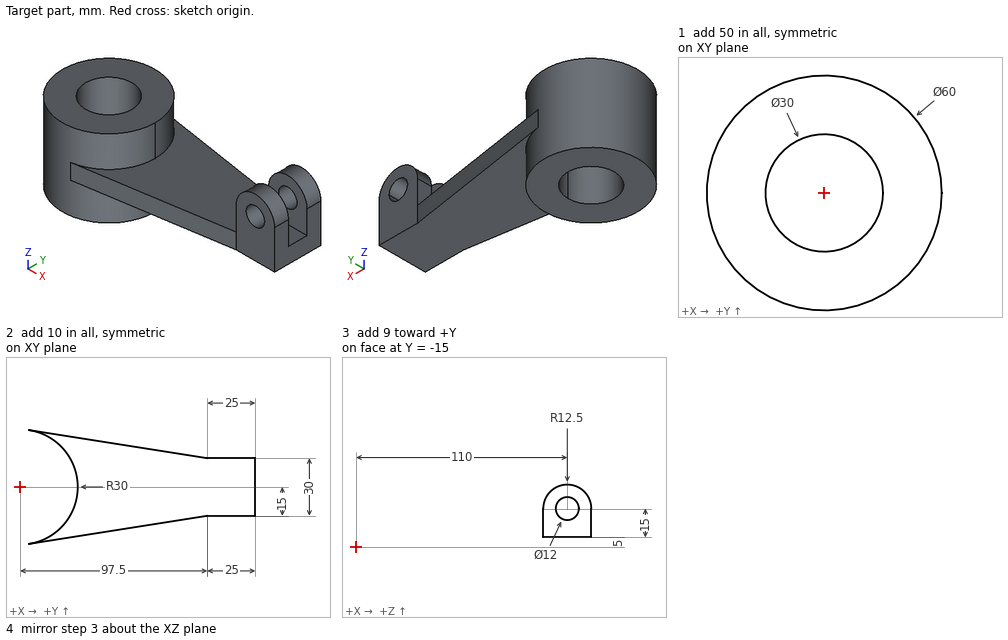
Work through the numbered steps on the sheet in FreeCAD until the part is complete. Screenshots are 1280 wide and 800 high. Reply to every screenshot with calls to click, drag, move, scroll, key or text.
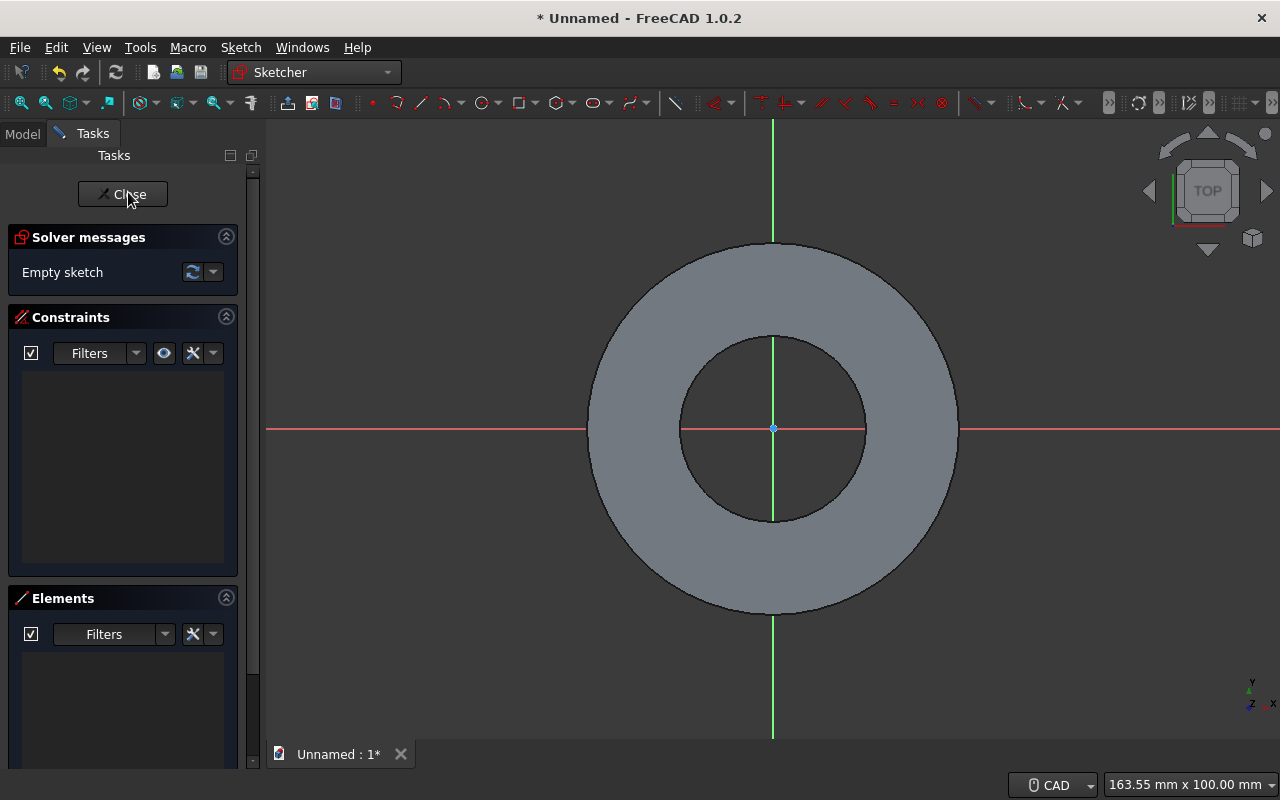
click(336, 104)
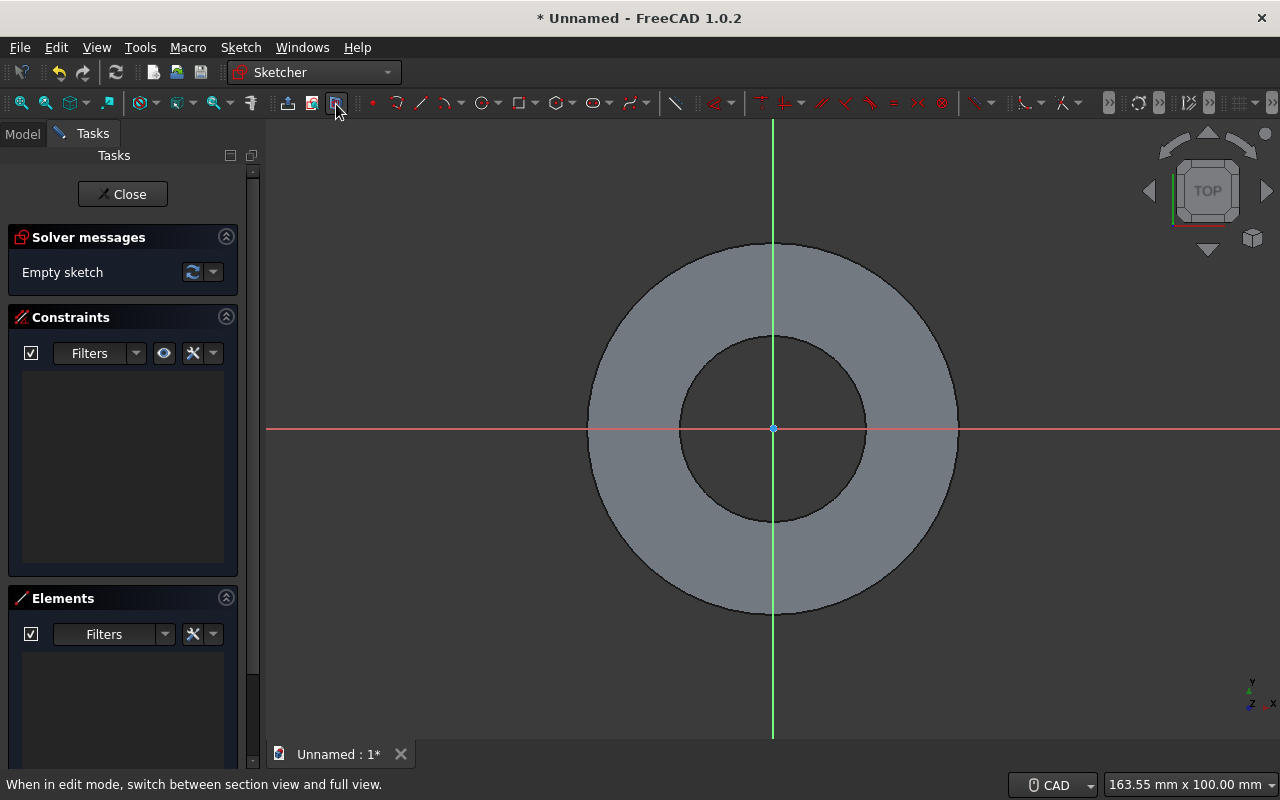
scroll(294, 429, down, 3)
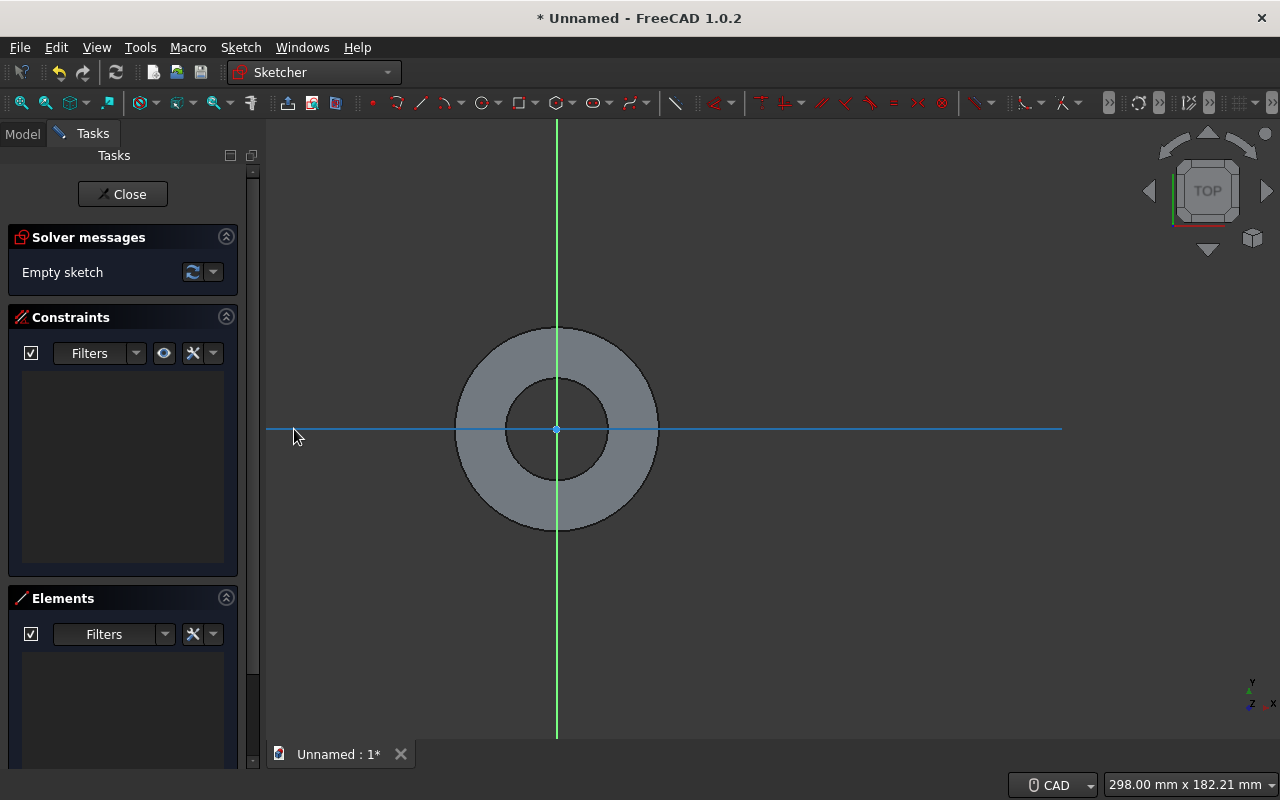
scroll(889, 430, up, 2)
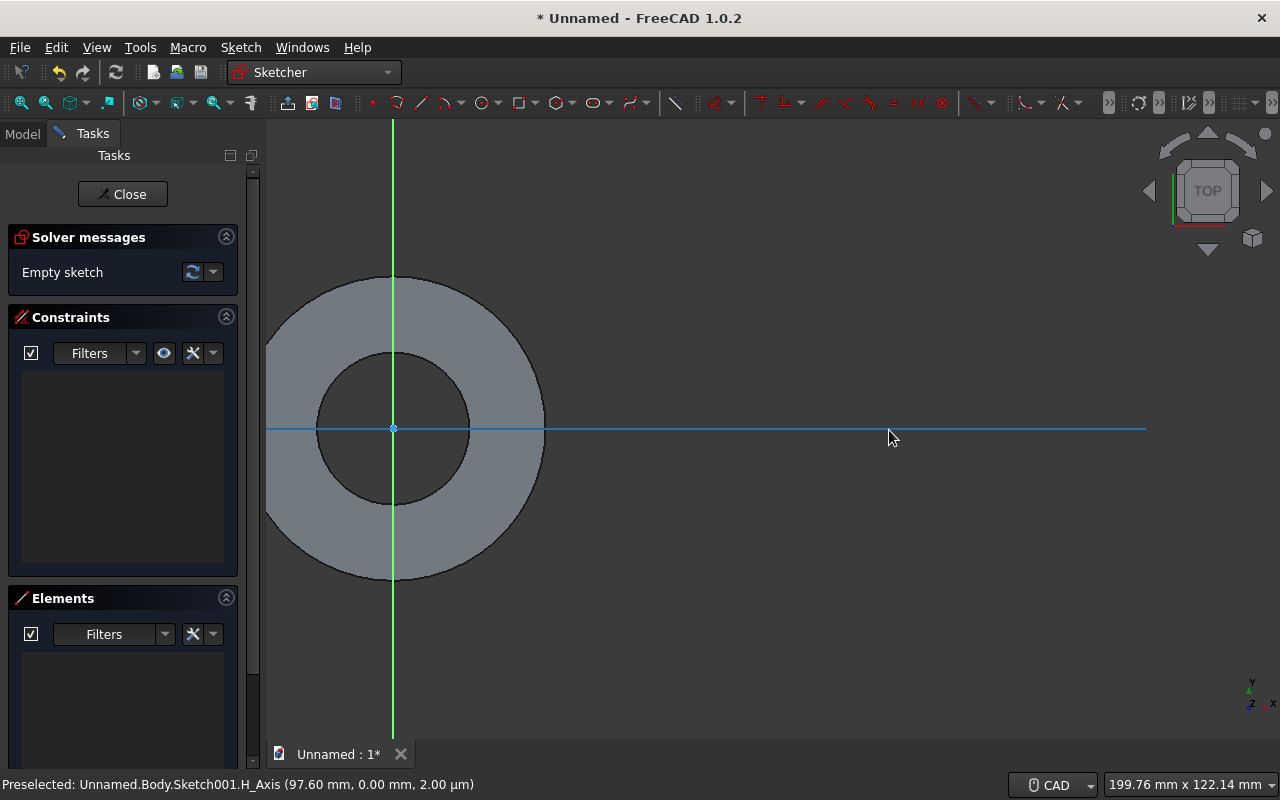
click(398, 104)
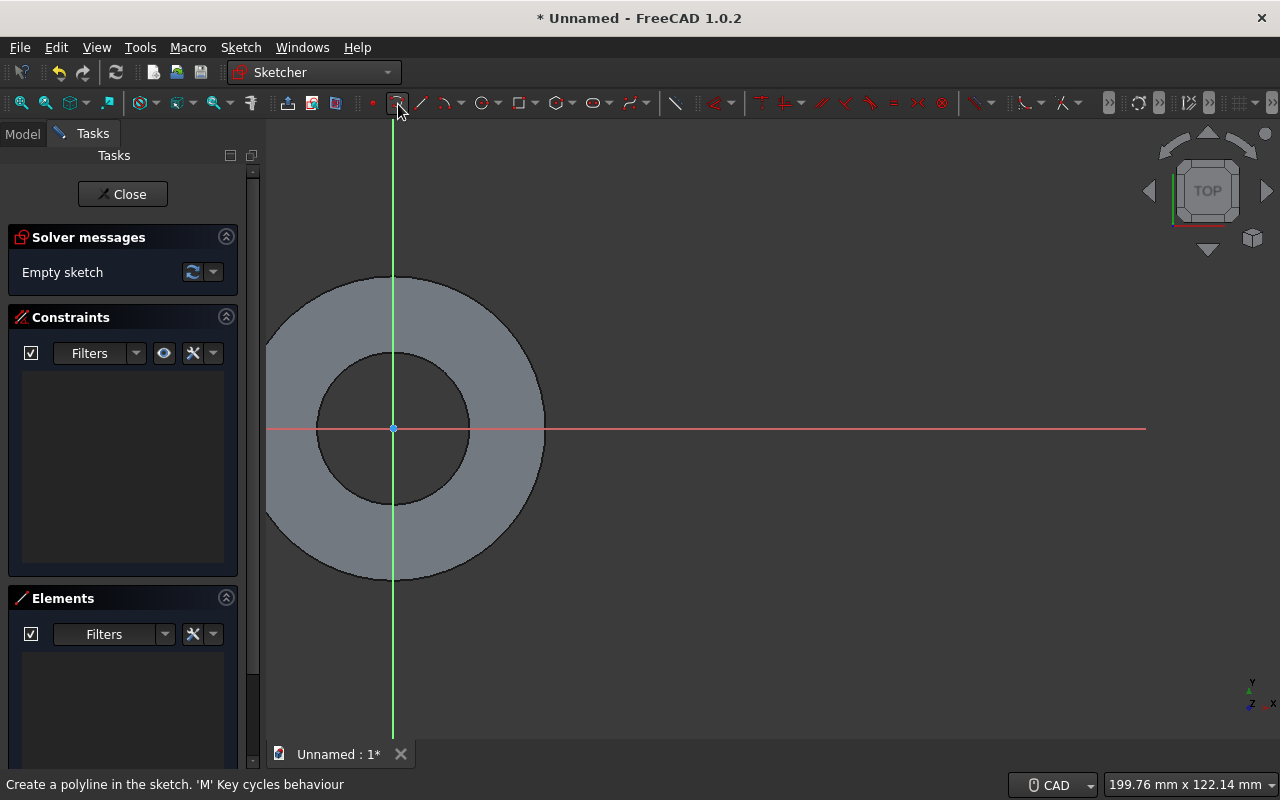
click(417, 579)
click(888, 505)
click(1015, 505)
click(1015, 352)
click(888, 352)
click(417, 278)
right_click(417, 278)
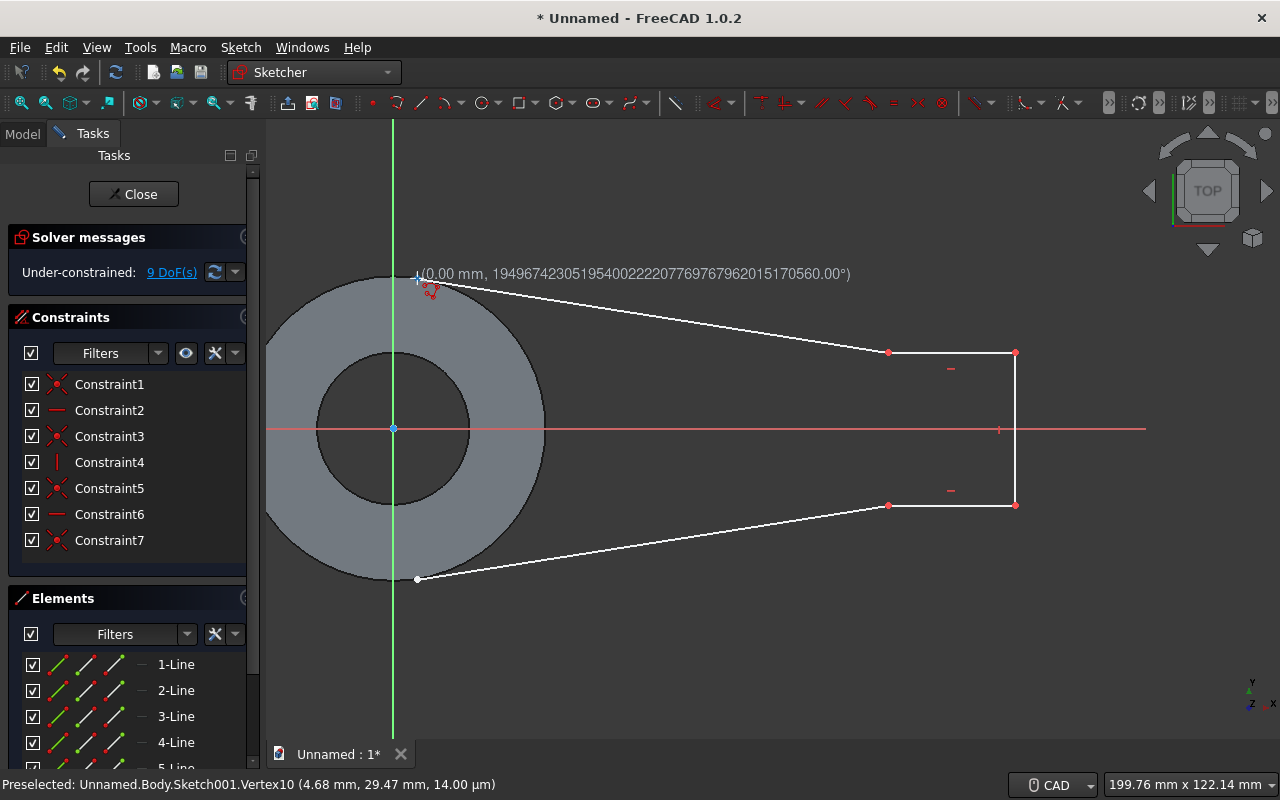
key(g)
key(3)
key(a)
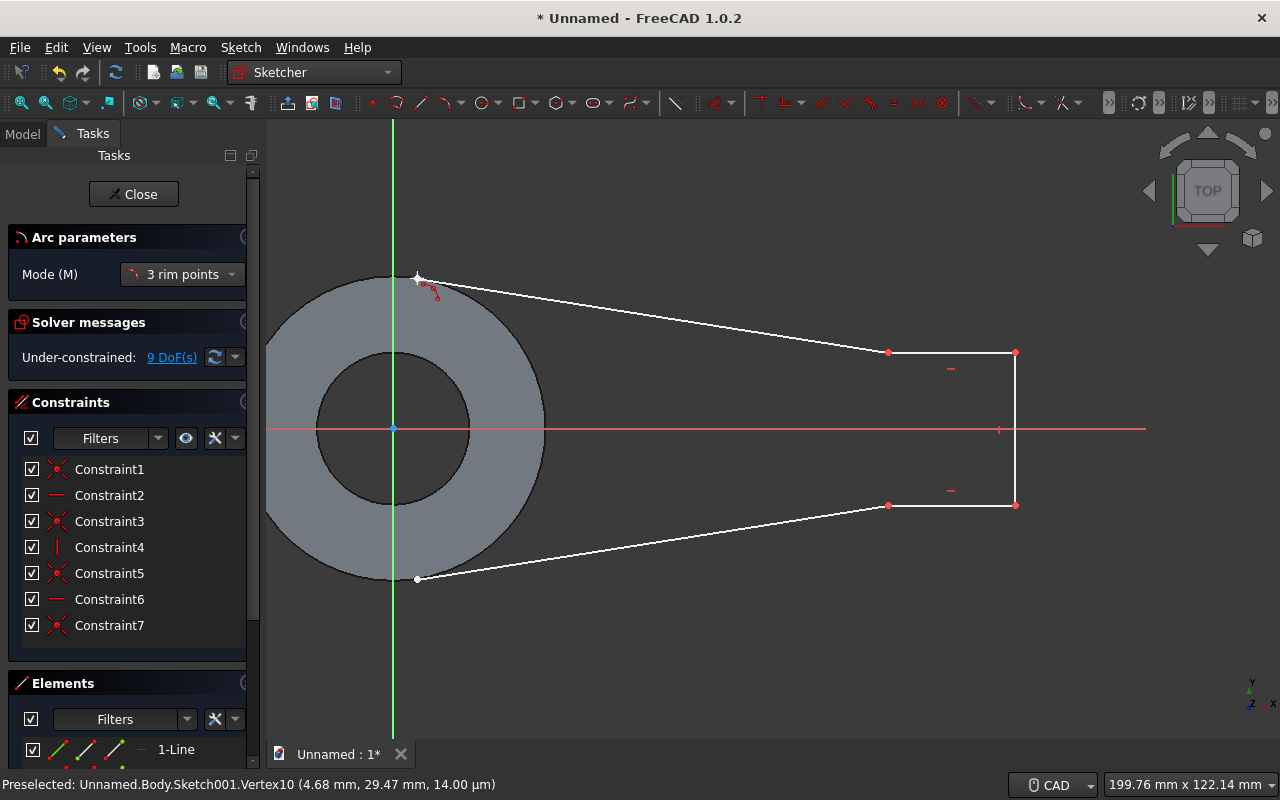
click(417, 279)
click(417, 580)
click(539, 471)
key(Escape)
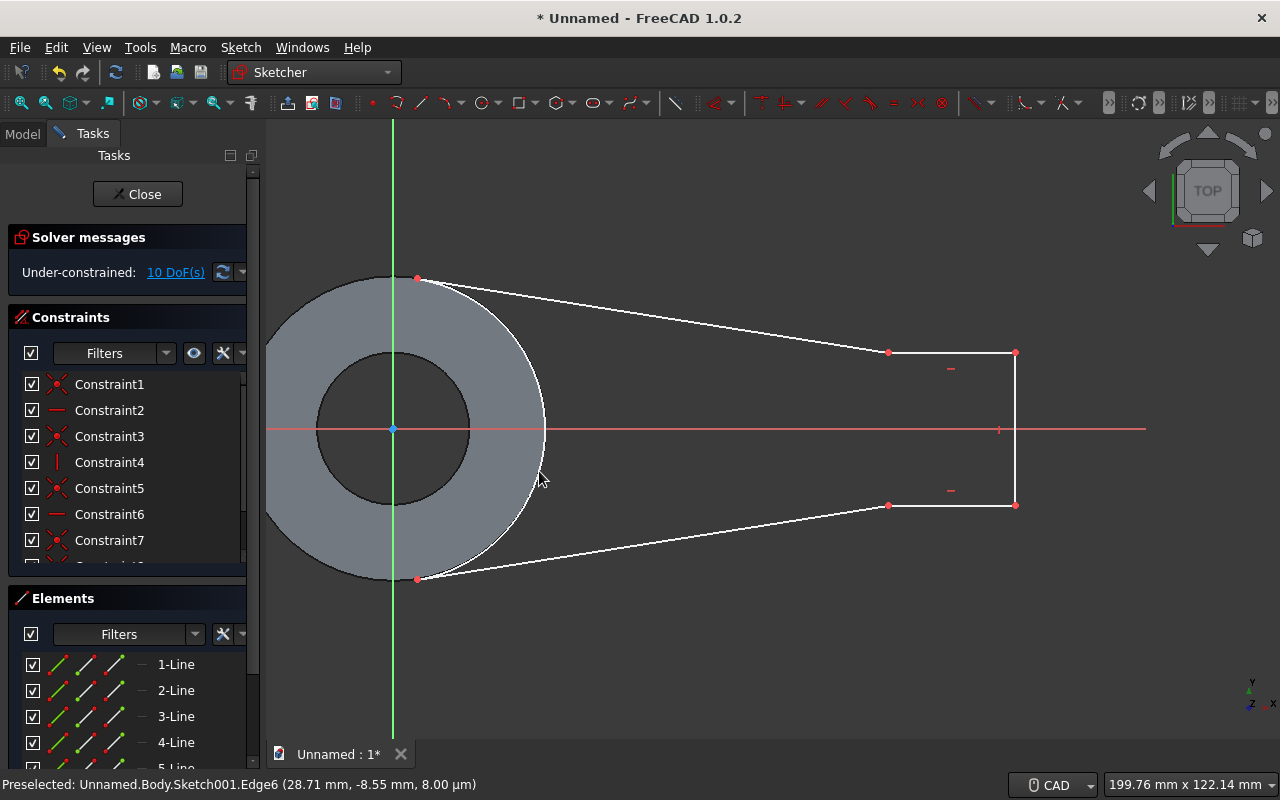
click(558, 558)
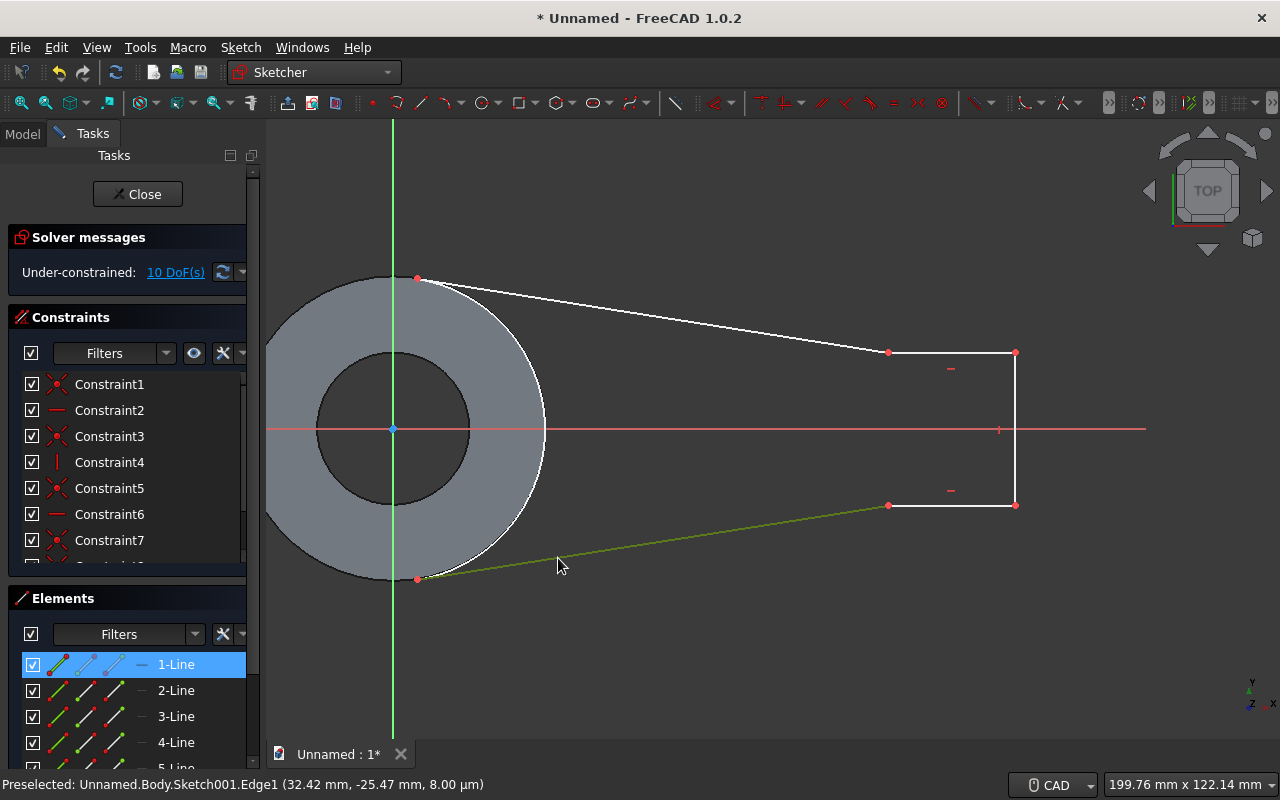
click(521, 511)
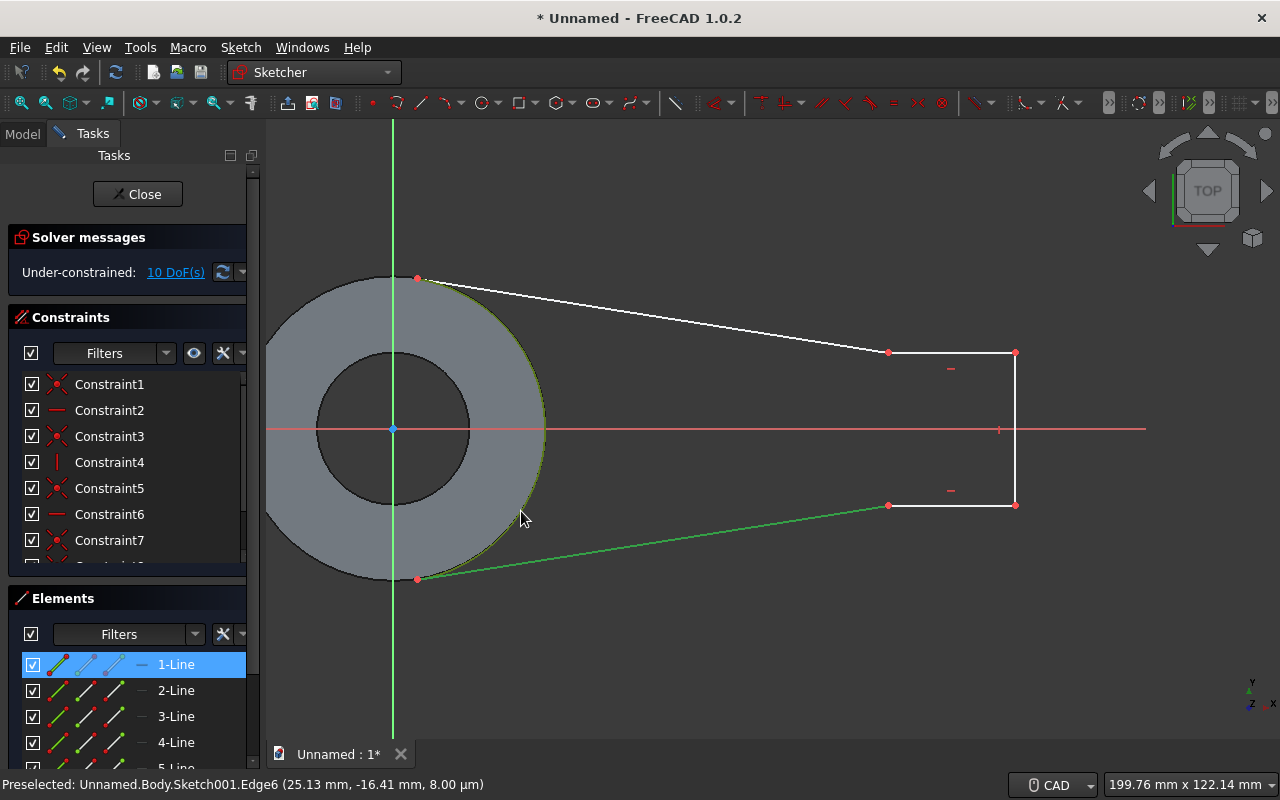
click(870, 104)